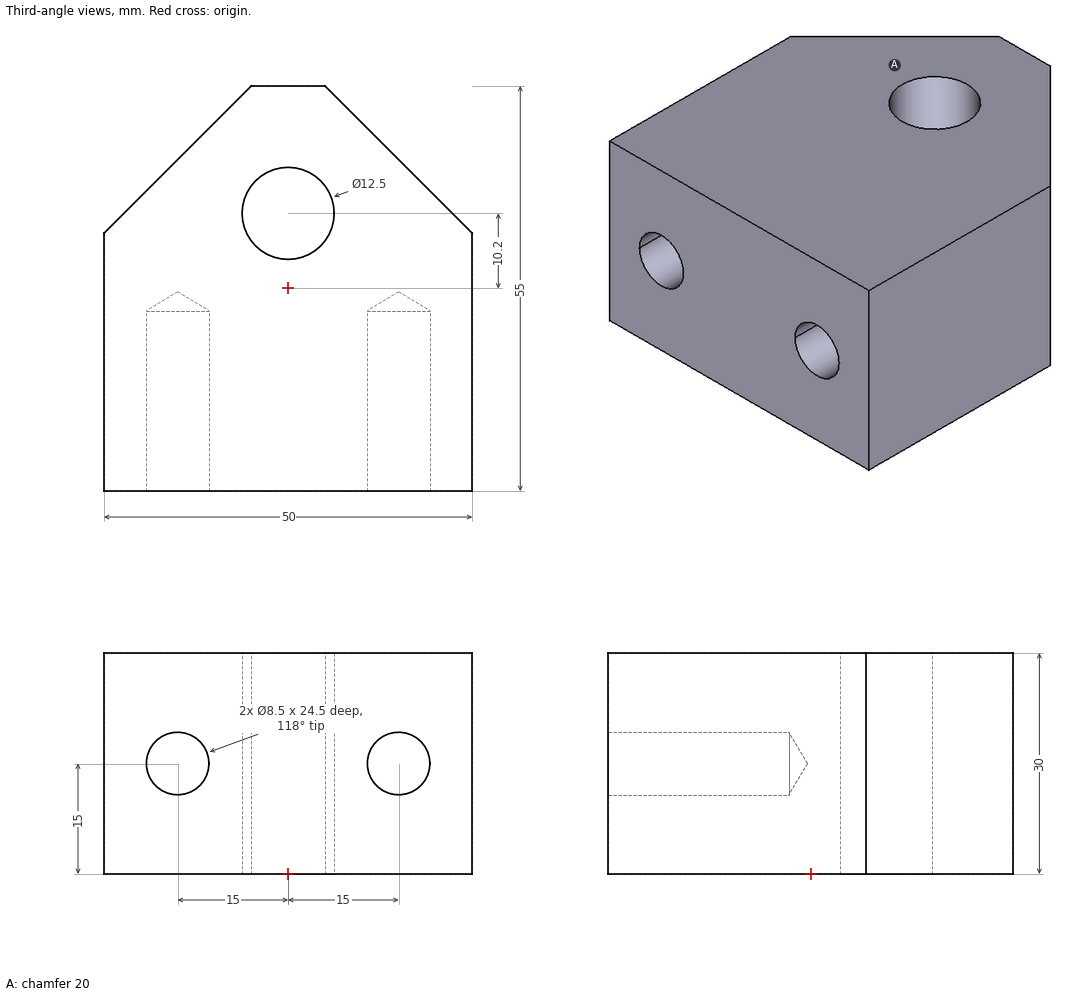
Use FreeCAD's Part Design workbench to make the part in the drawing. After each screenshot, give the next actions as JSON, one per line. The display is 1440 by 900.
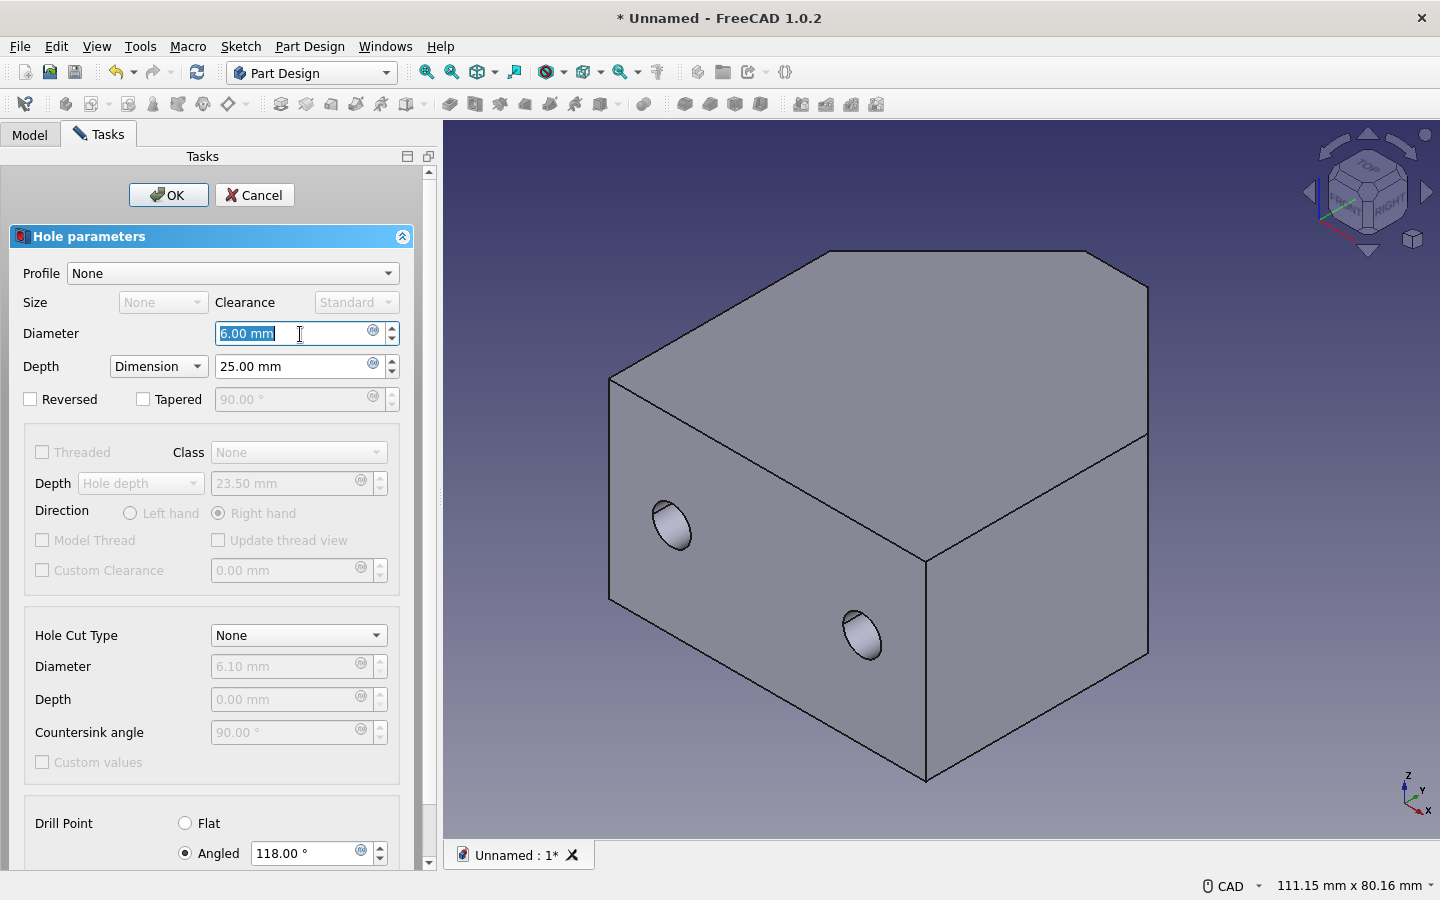
{"action": "type", "text": "8.5"}
{"action": "key", "text": "Tab"}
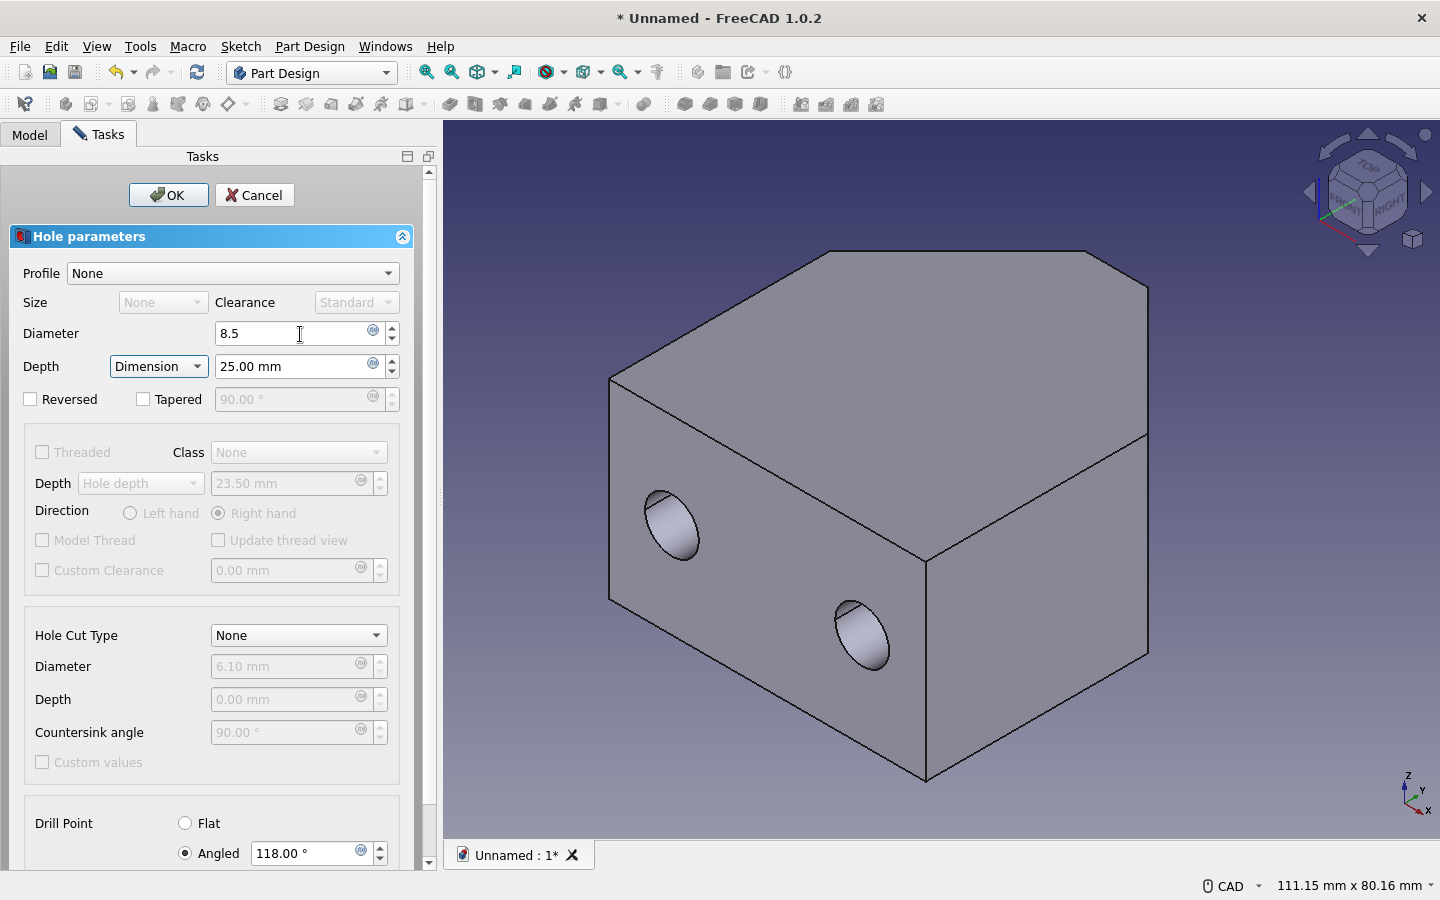
{"action": "triple_click", "coordinate": [300, 366]}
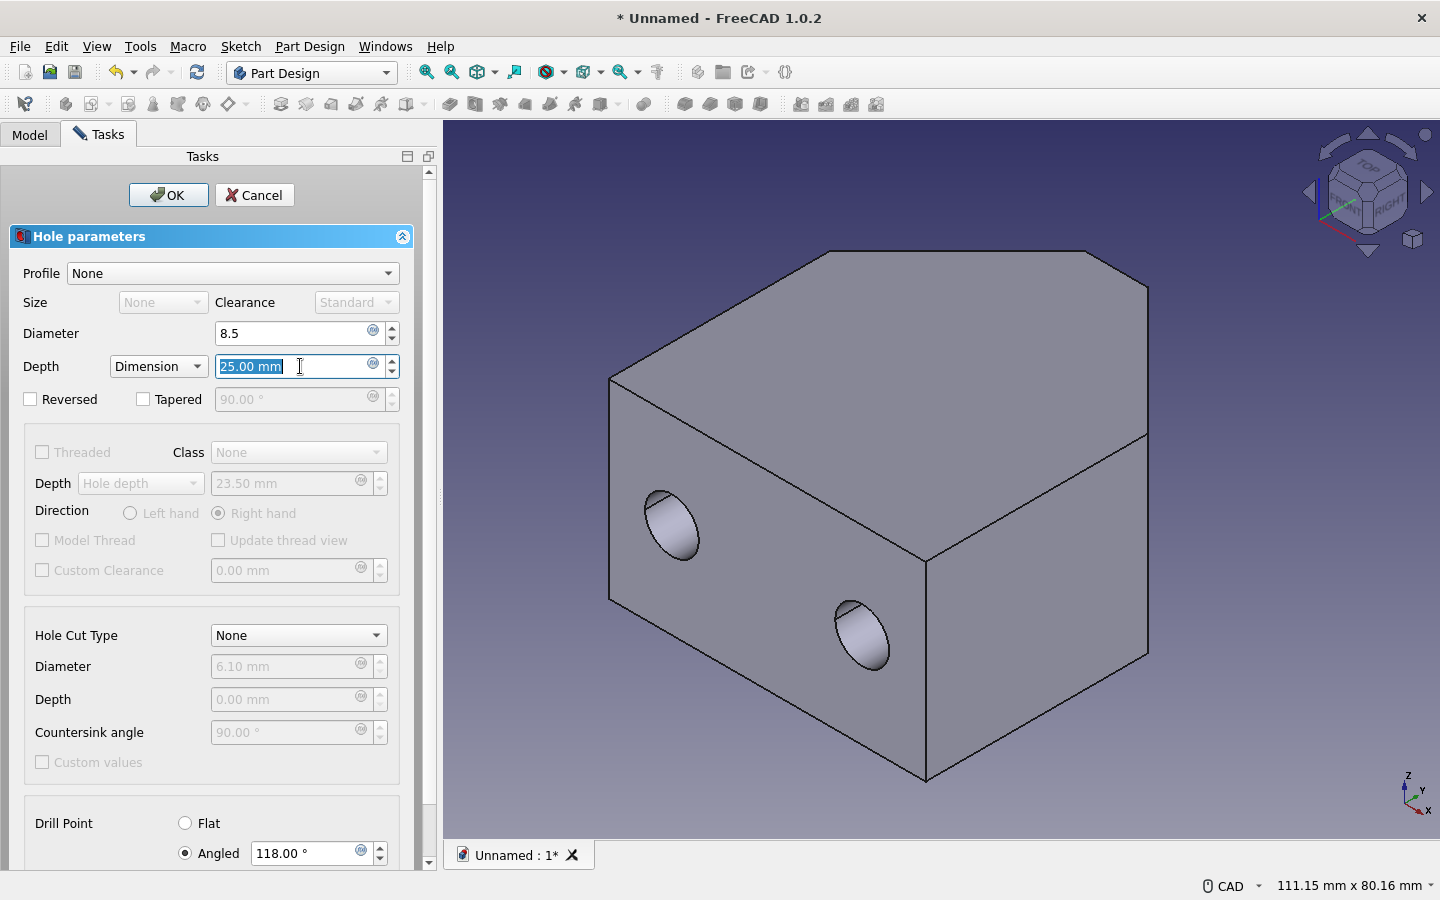
{"action": "type", "text": "24.5"}
{"action": "key", "text": "Tab"}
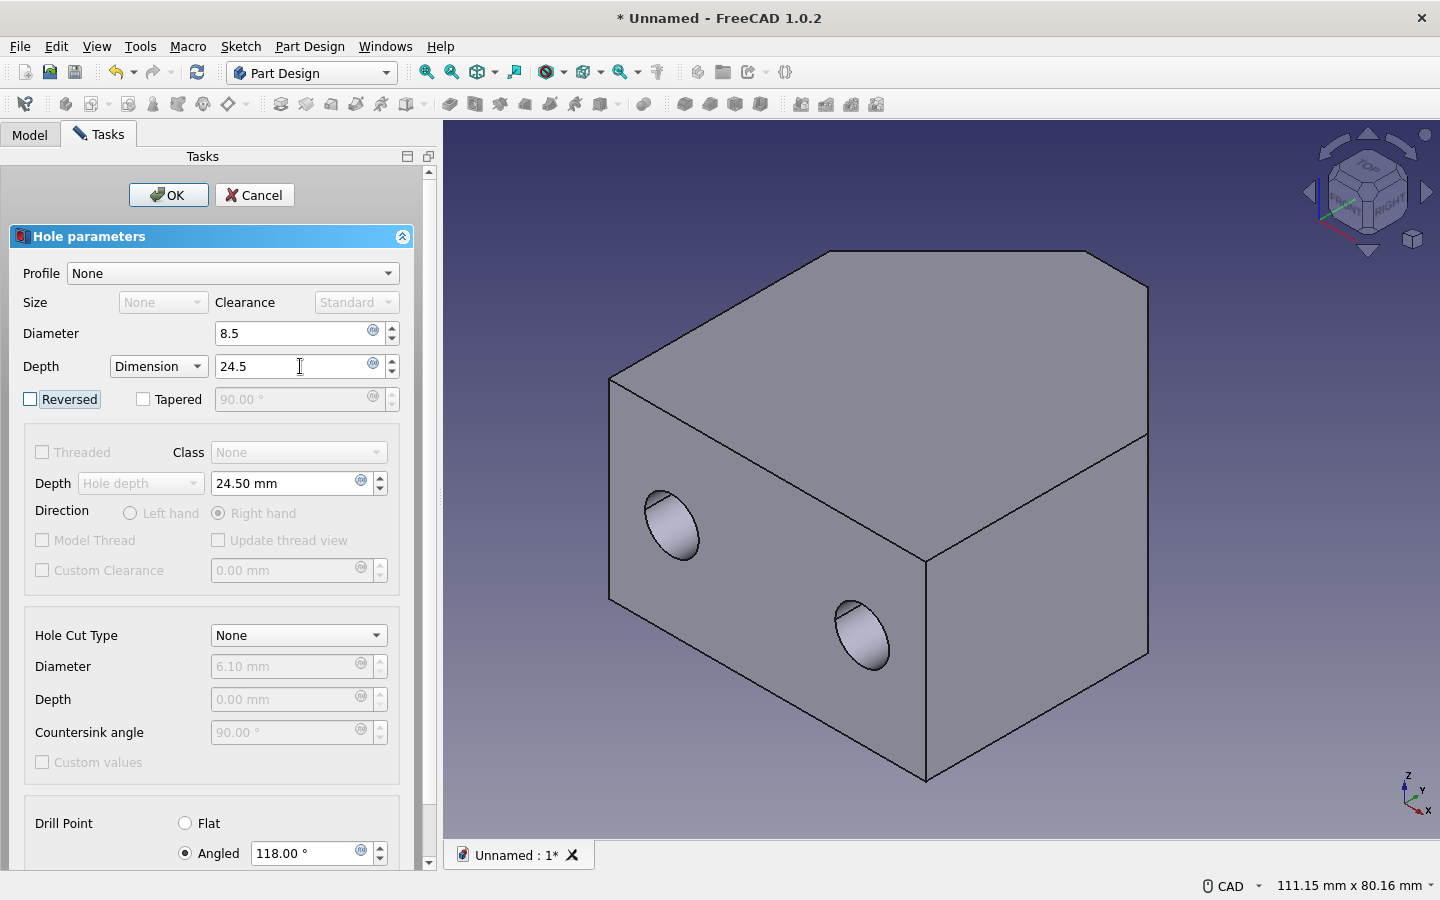
{"action": "left_click", "coordinate": [169, 195]}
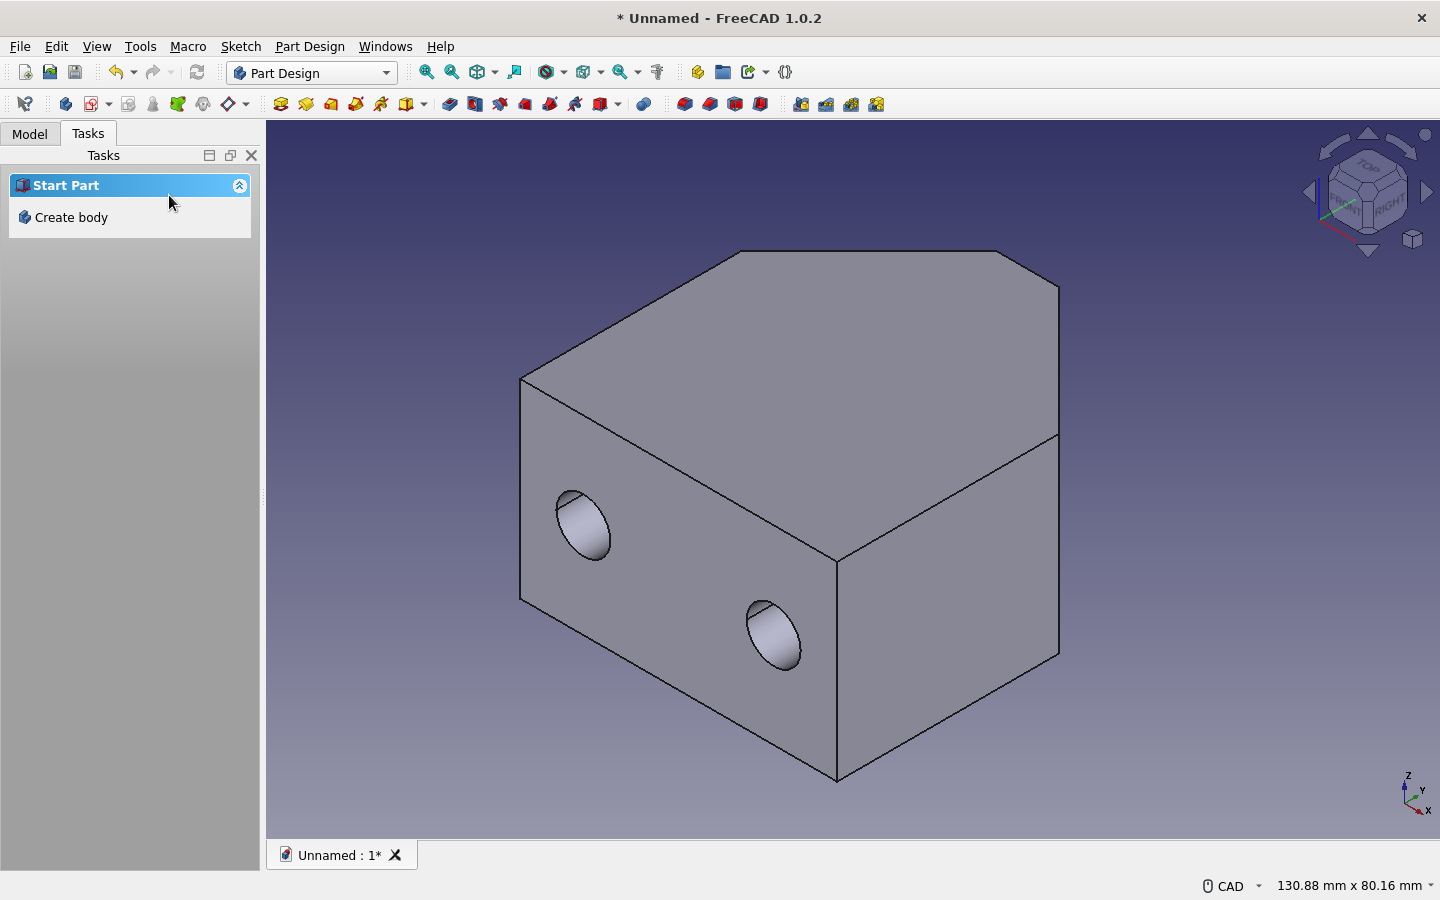
{"action": "left_click", "coordinate": [853, 369]}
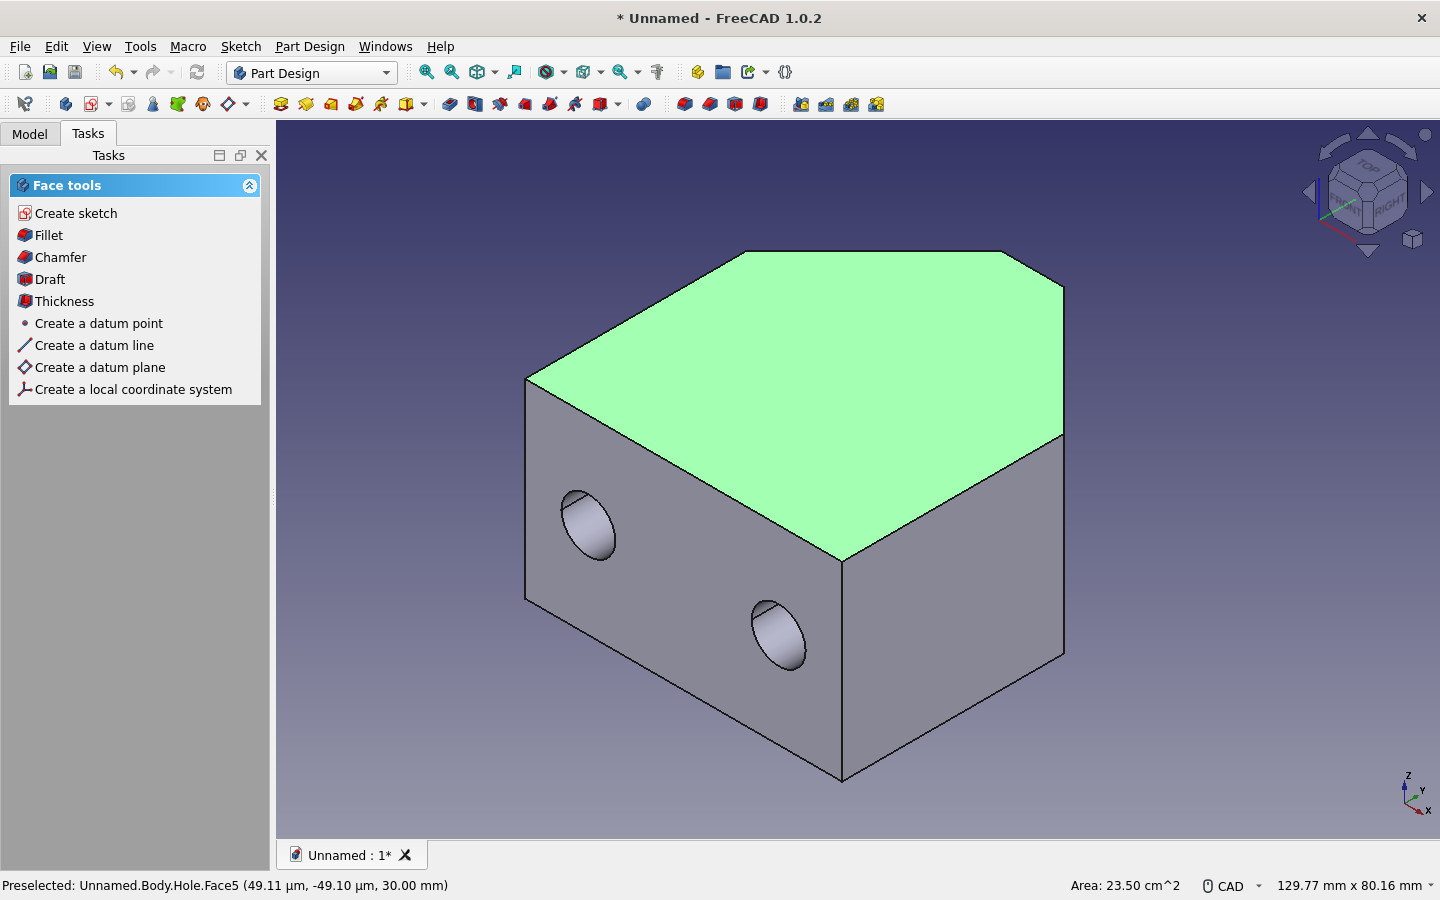
{"action": "left_click", "coordinate": [90, 104]}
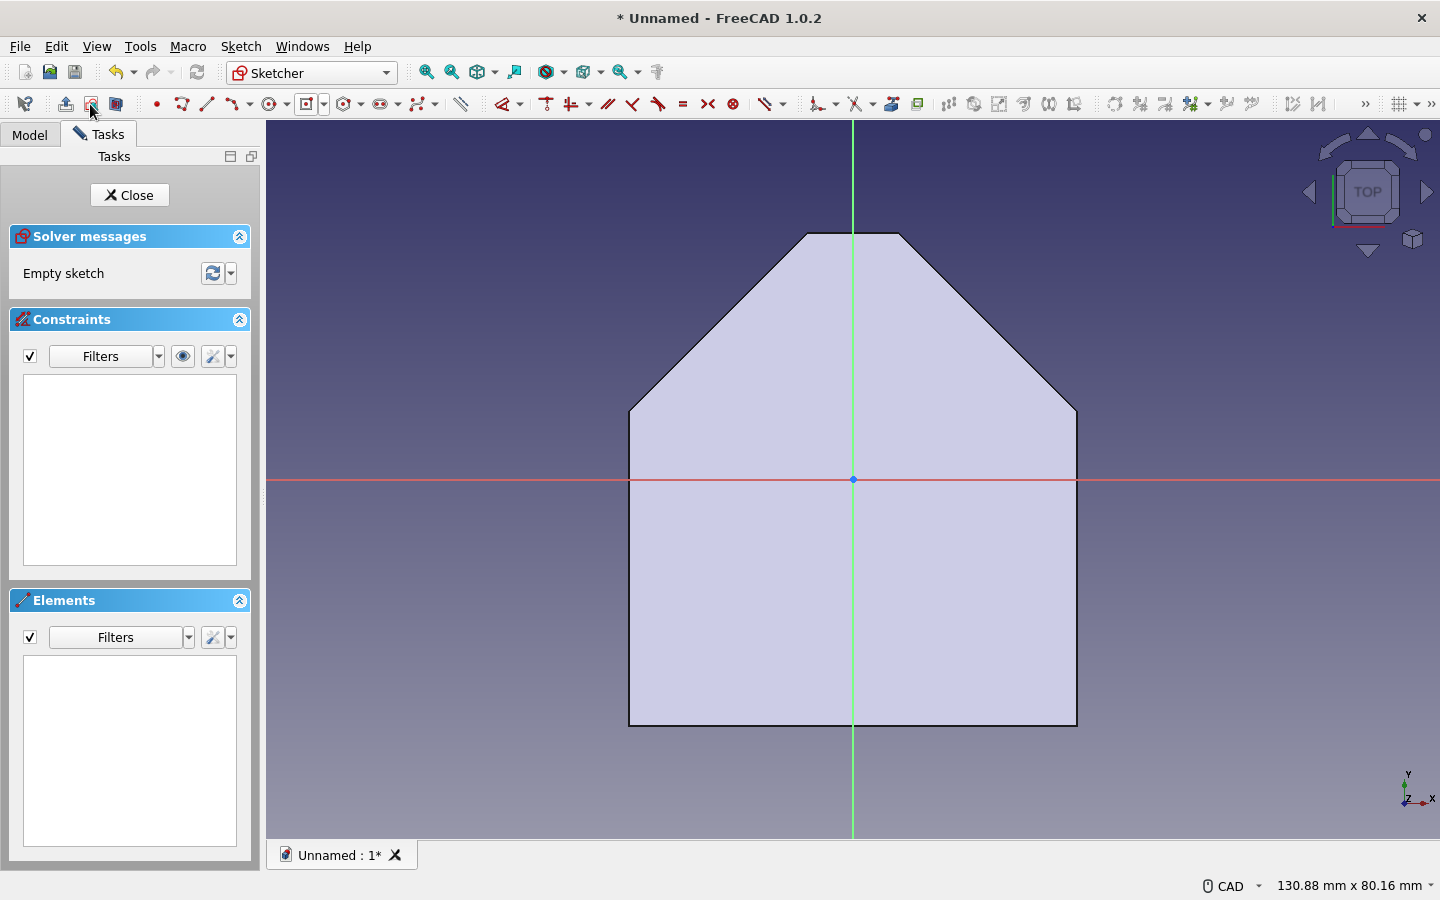
{"action": "scroll", "coordinate": [883, 374], "scroll_direction": "up", "scroll_amount": 6}